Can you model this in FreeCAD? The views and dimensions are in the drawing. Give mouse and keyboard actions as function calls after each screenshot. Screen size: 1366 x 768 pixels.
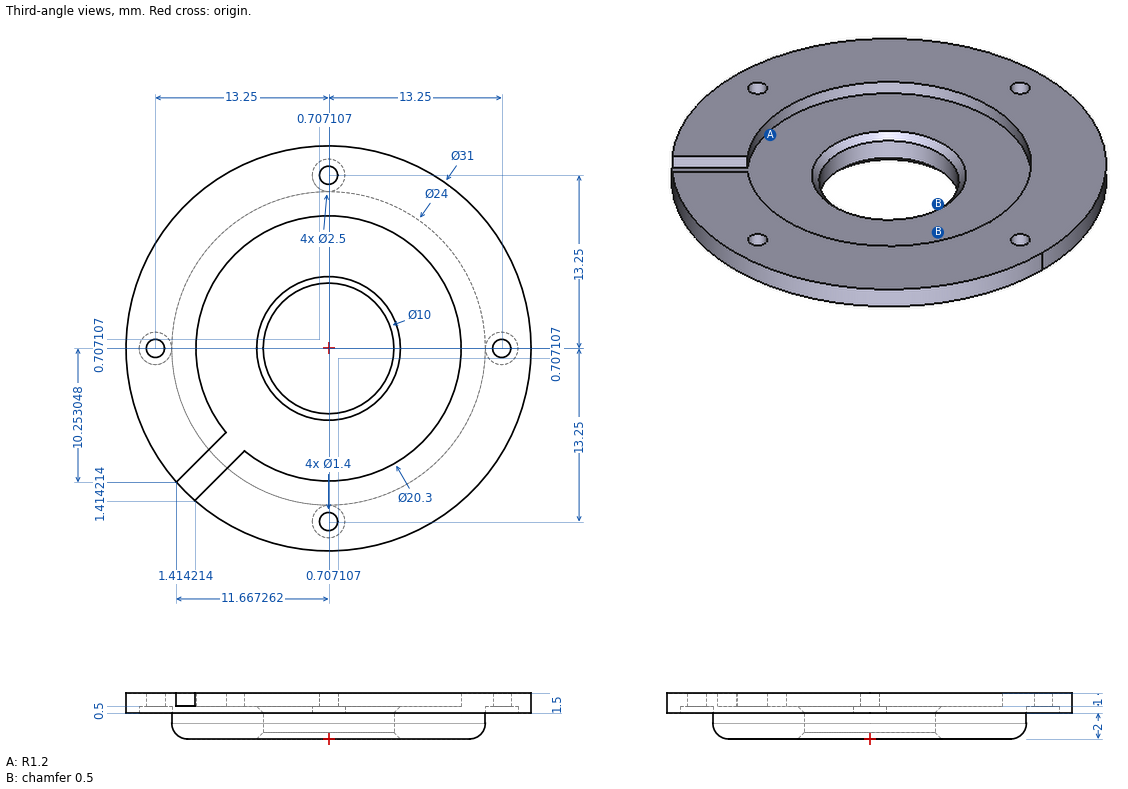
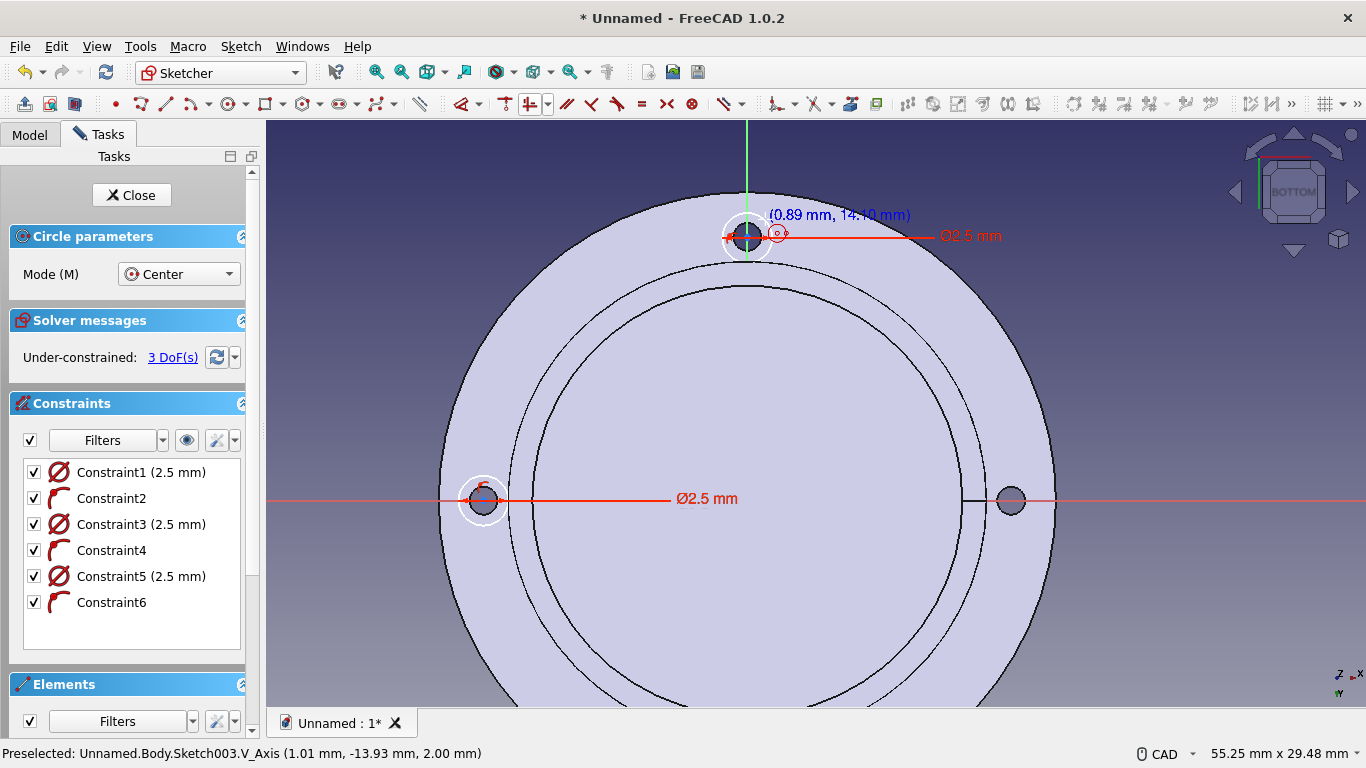
click(1011, 501)
move(1029, 483)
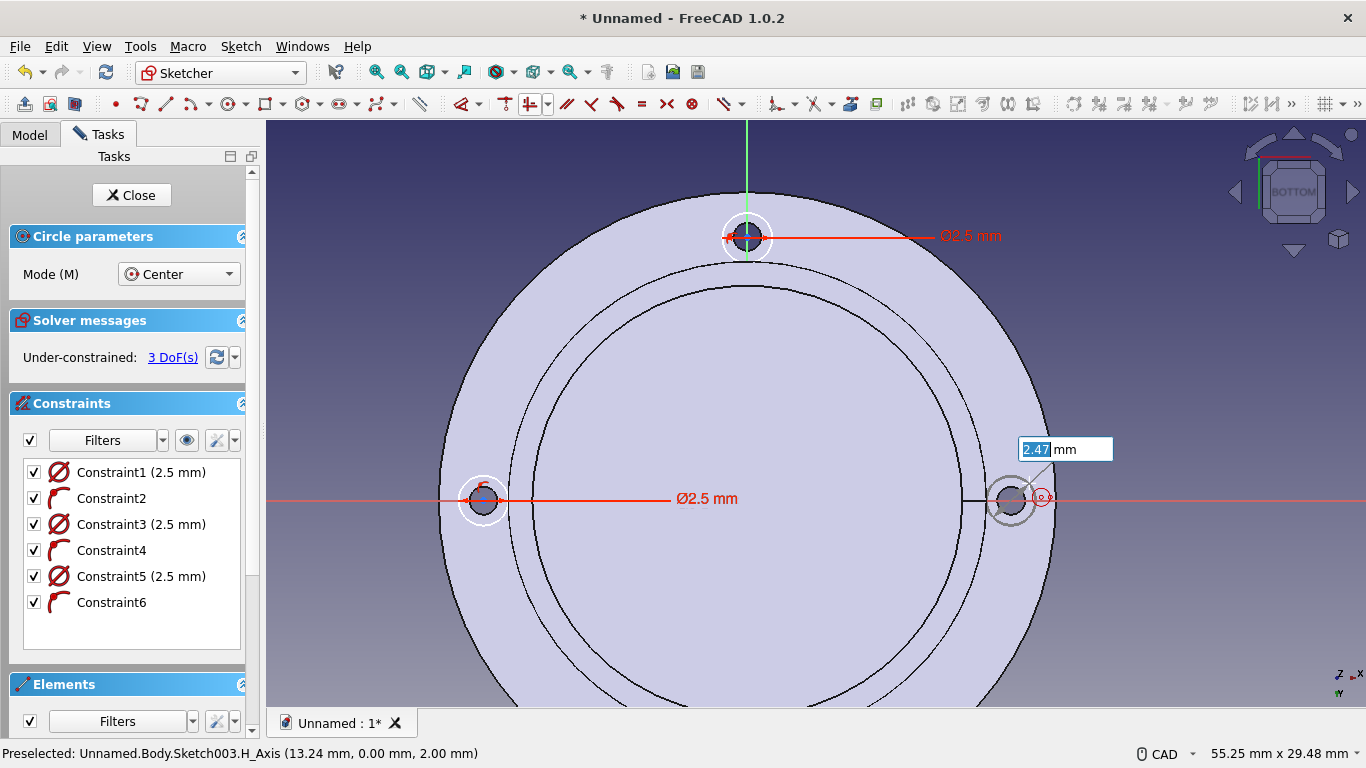
text(2.5)
key(Return)
key(Escape)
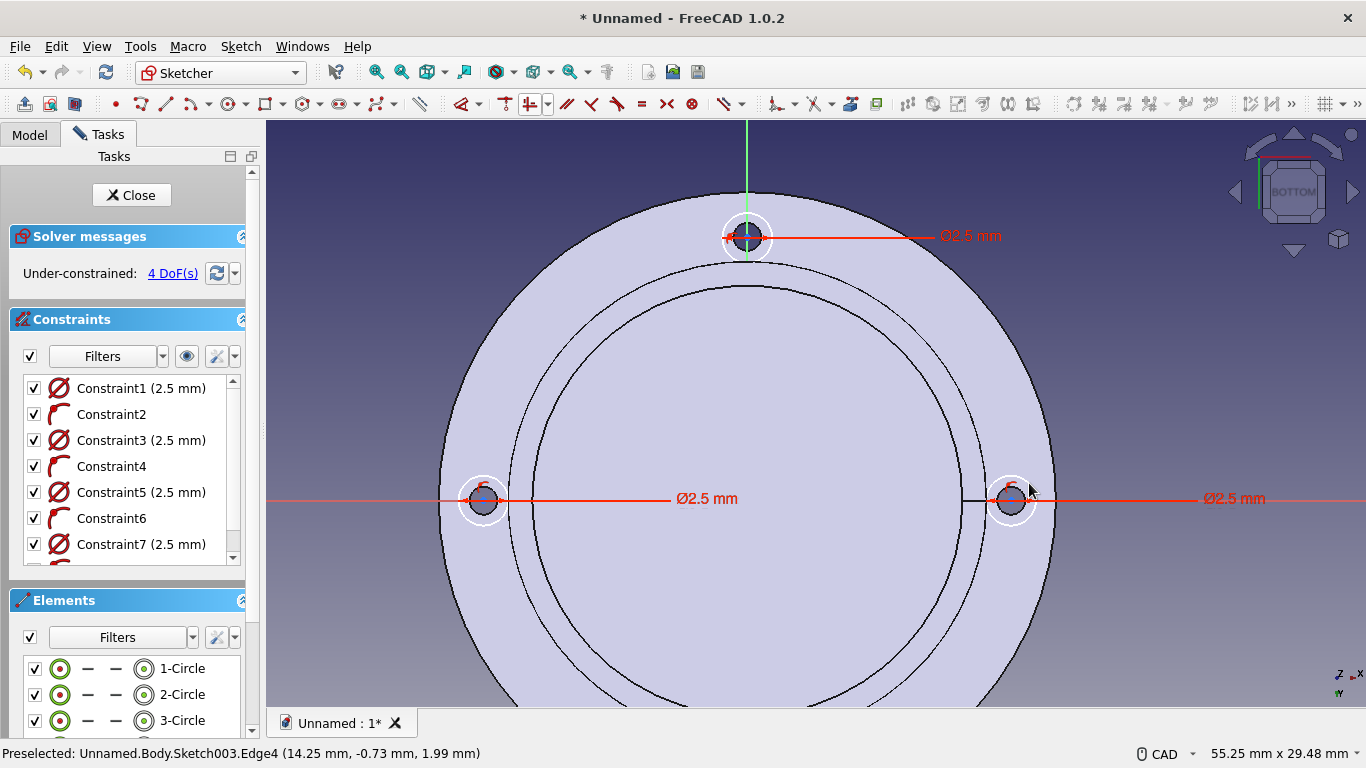
click(460, 104)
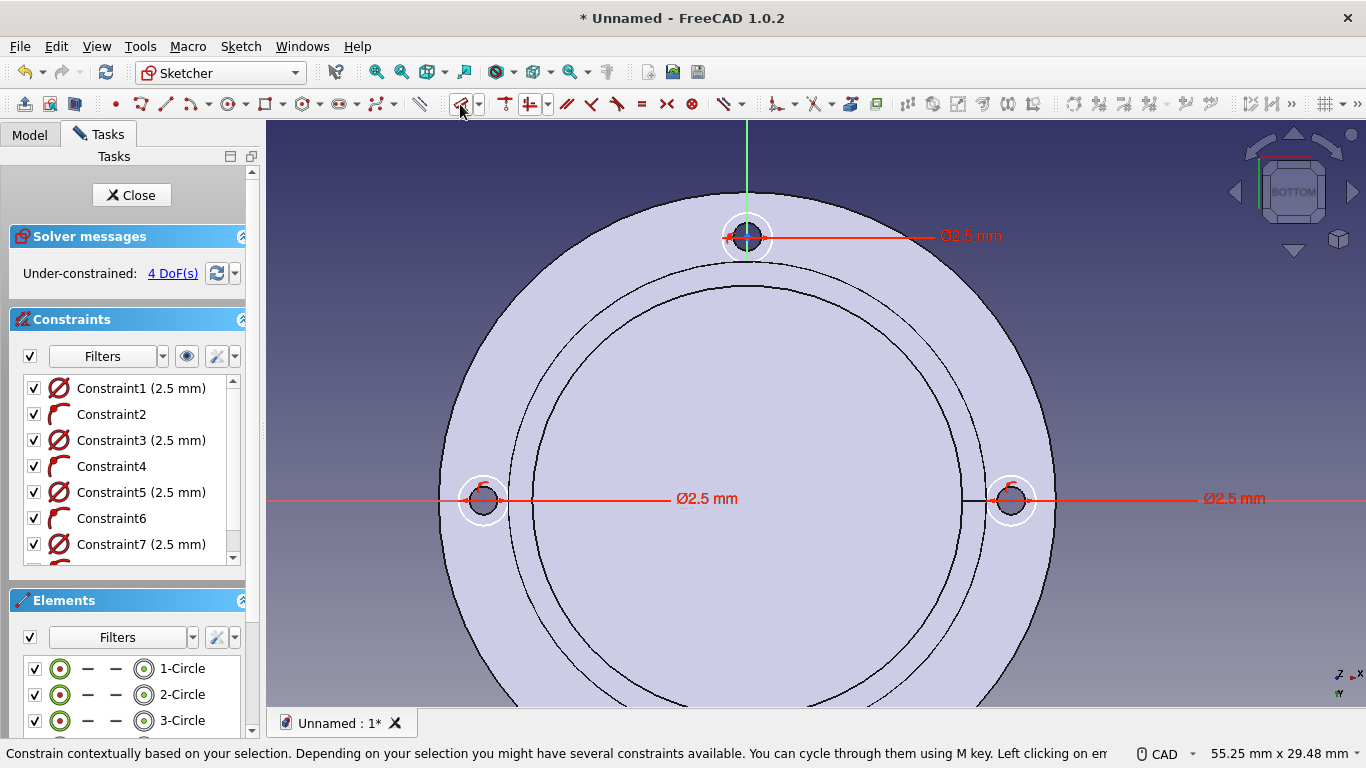
scroll(748, 236, down, 2)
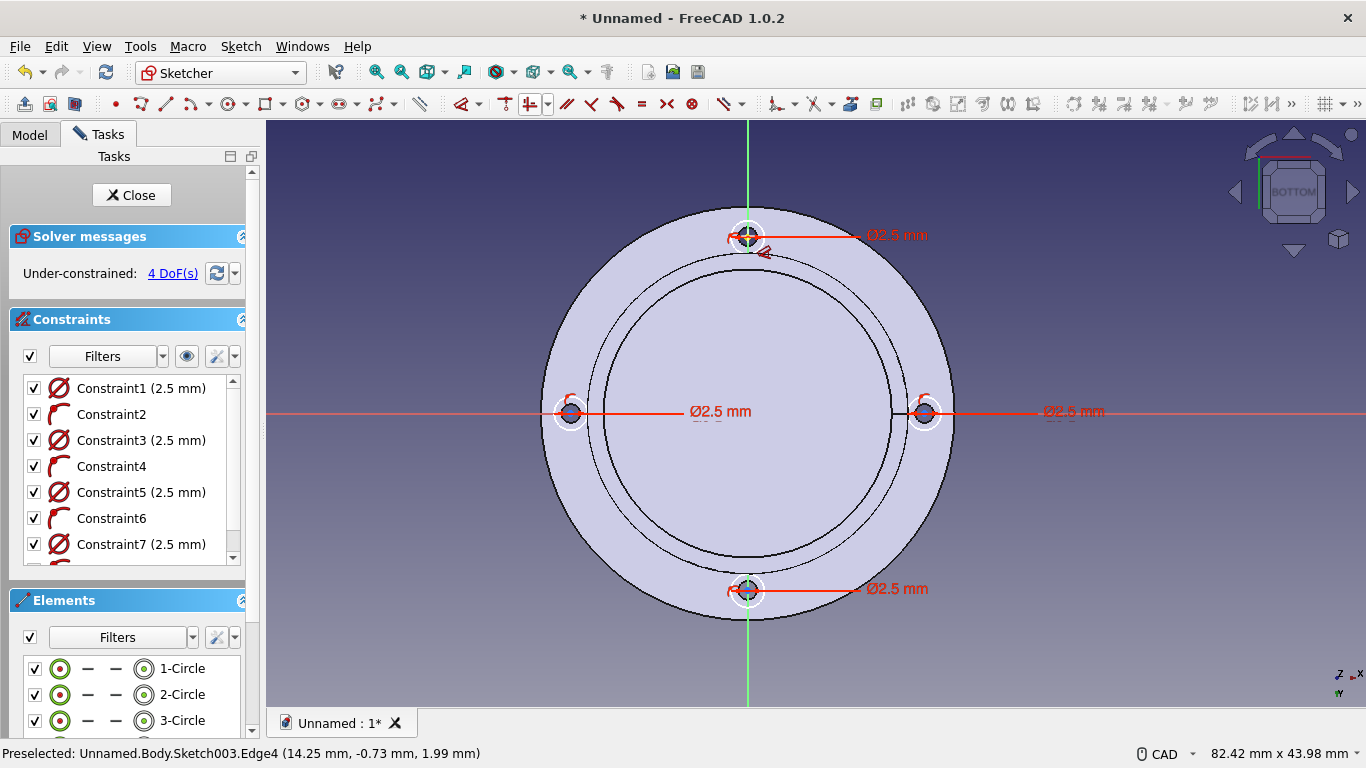
click(748, 591)
click(782, 502)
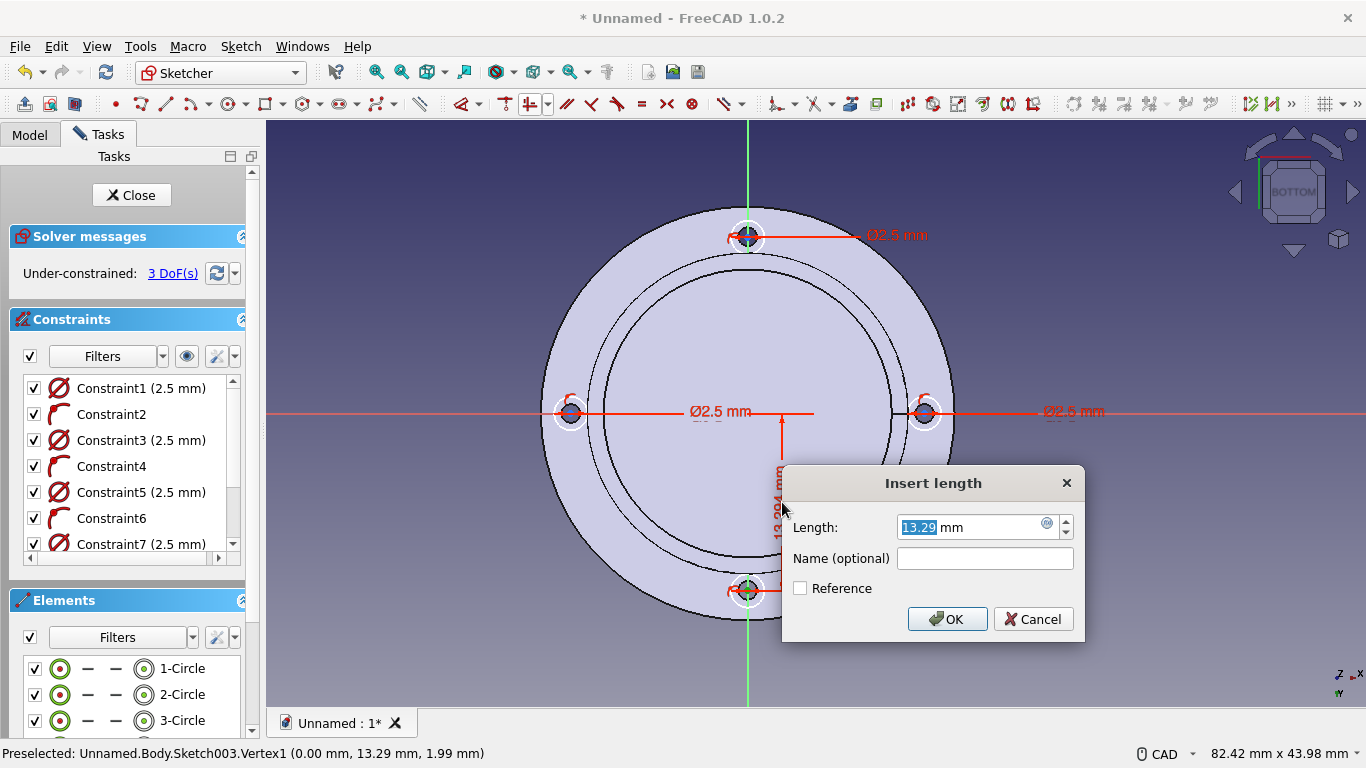
text(13.25)
key(Return)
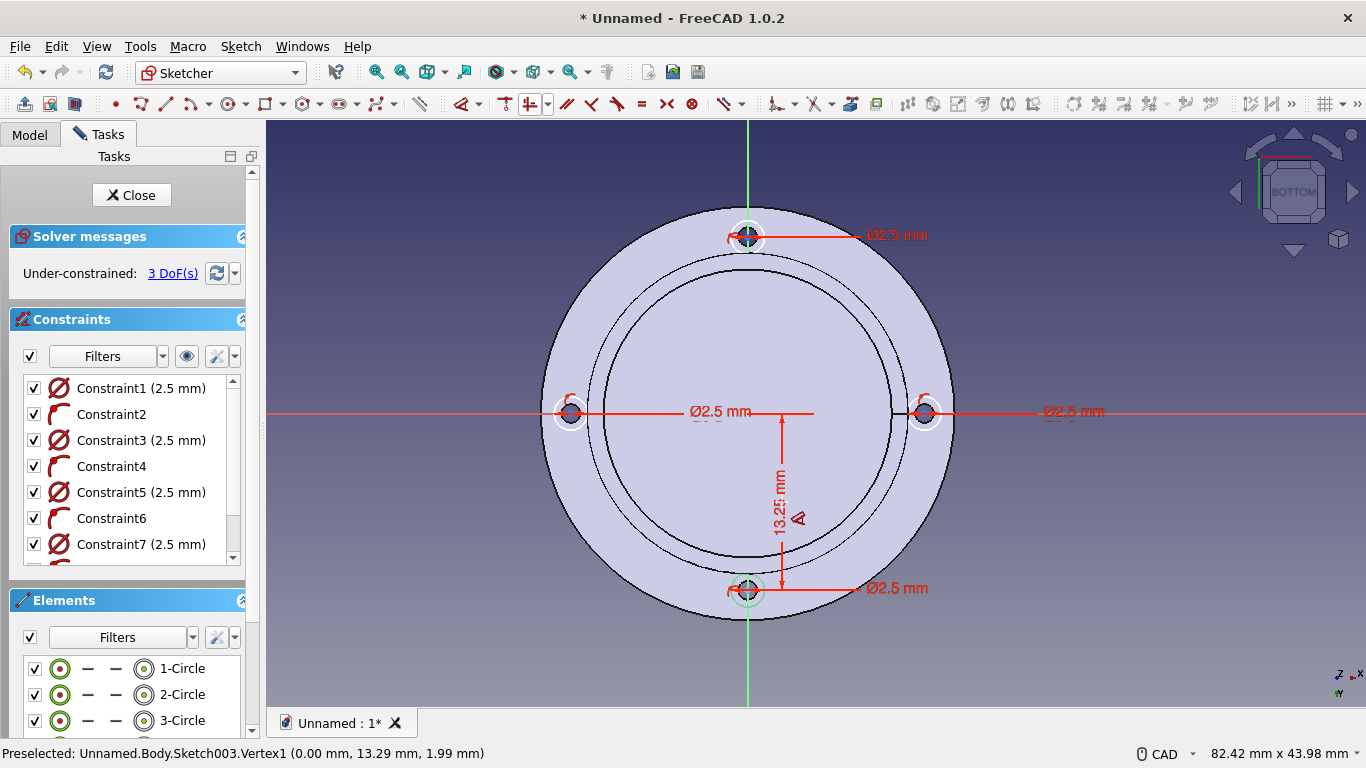
click(571, 414)
click(659, 448)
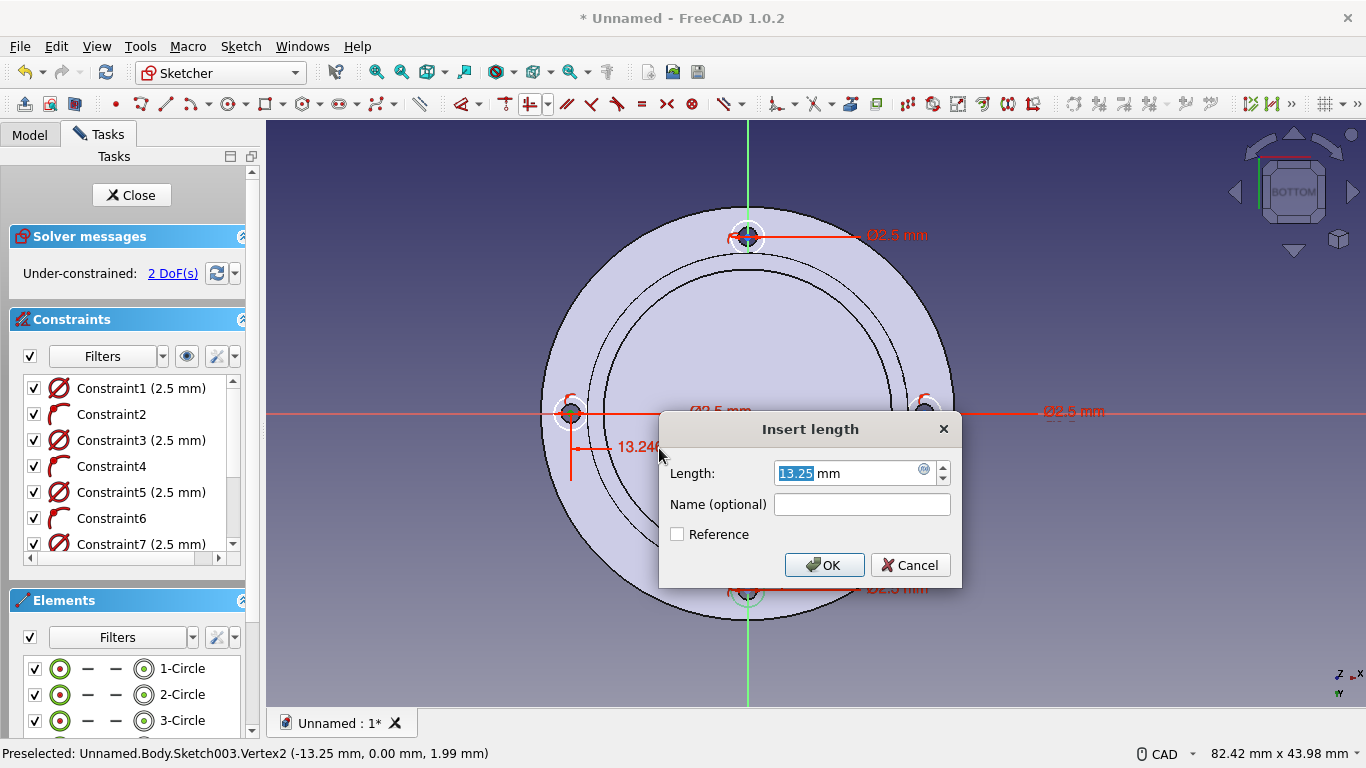
text(13.25)
key(Return)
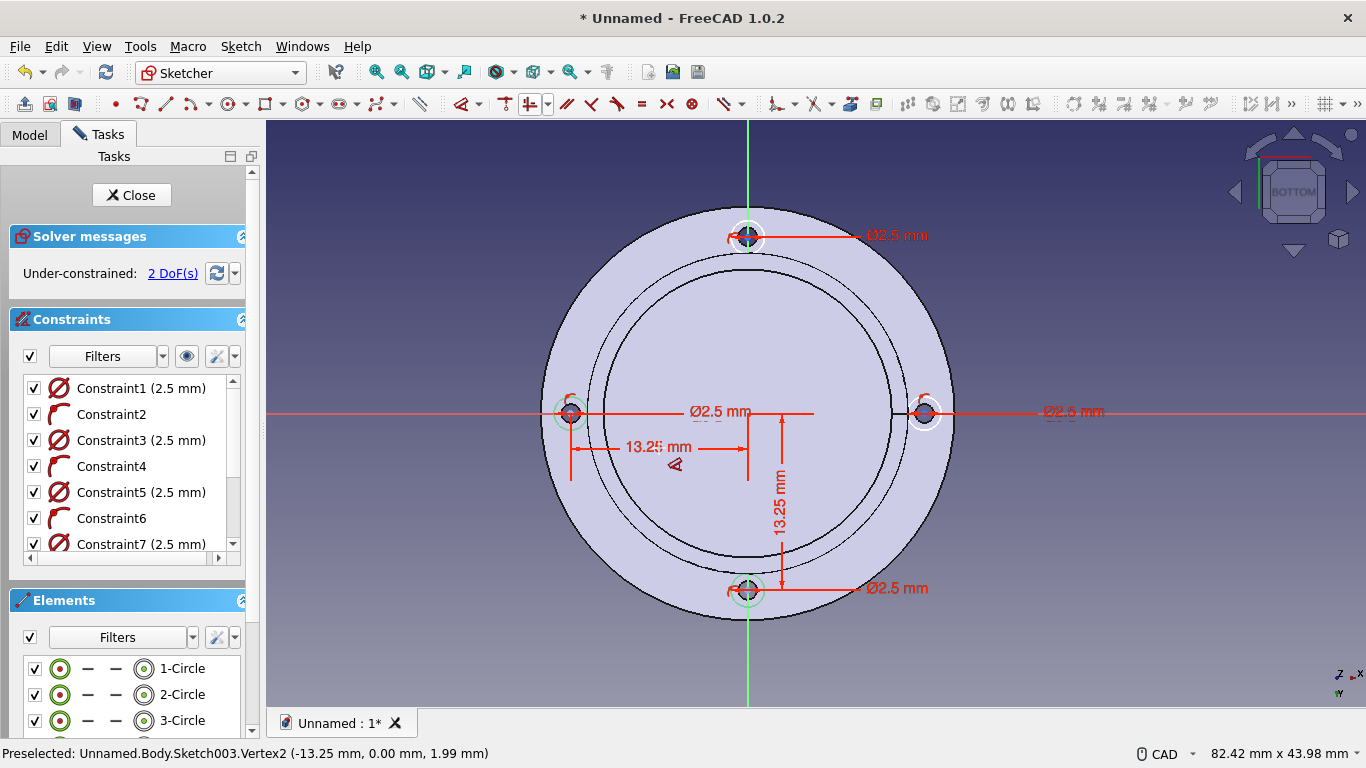
click(748, 237)
click(782, 325)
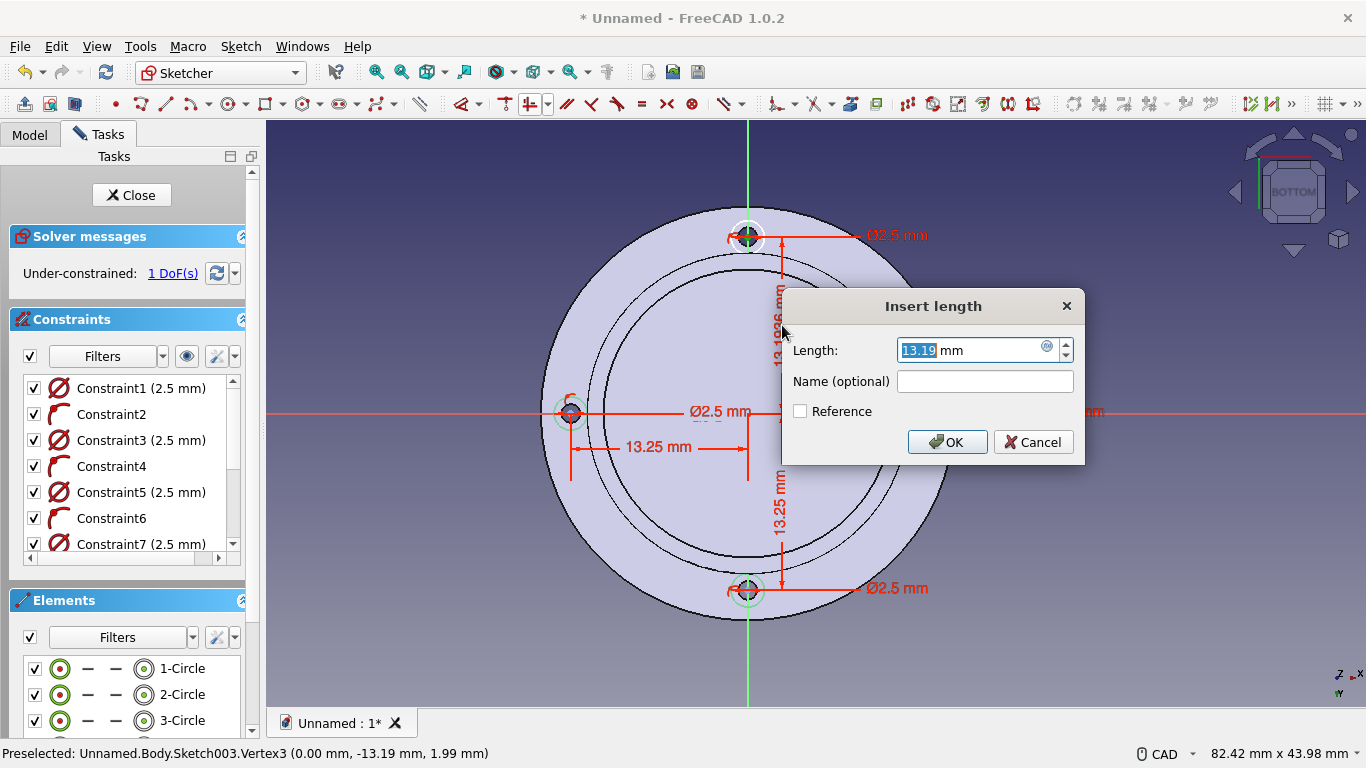
text(13.25)
key(Return)